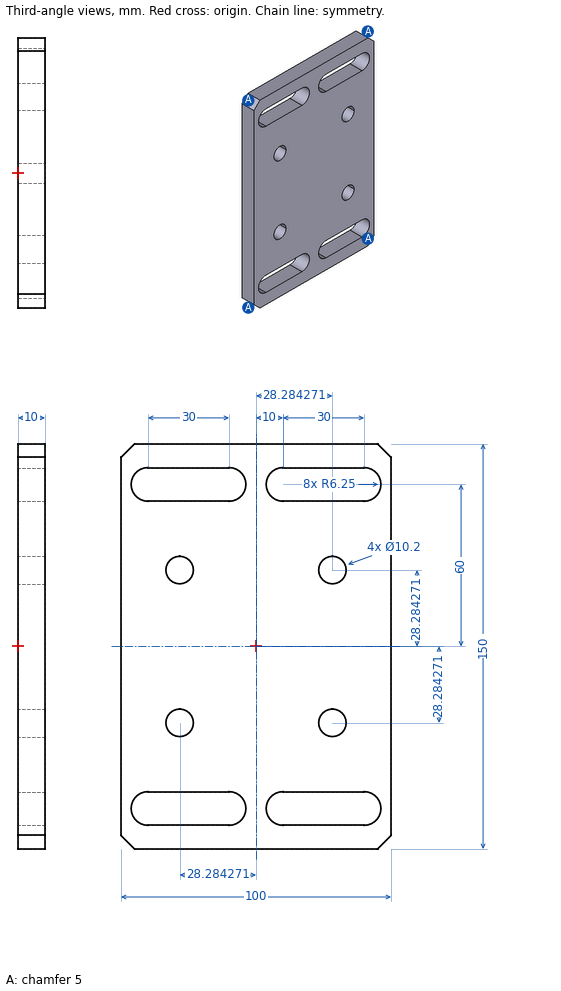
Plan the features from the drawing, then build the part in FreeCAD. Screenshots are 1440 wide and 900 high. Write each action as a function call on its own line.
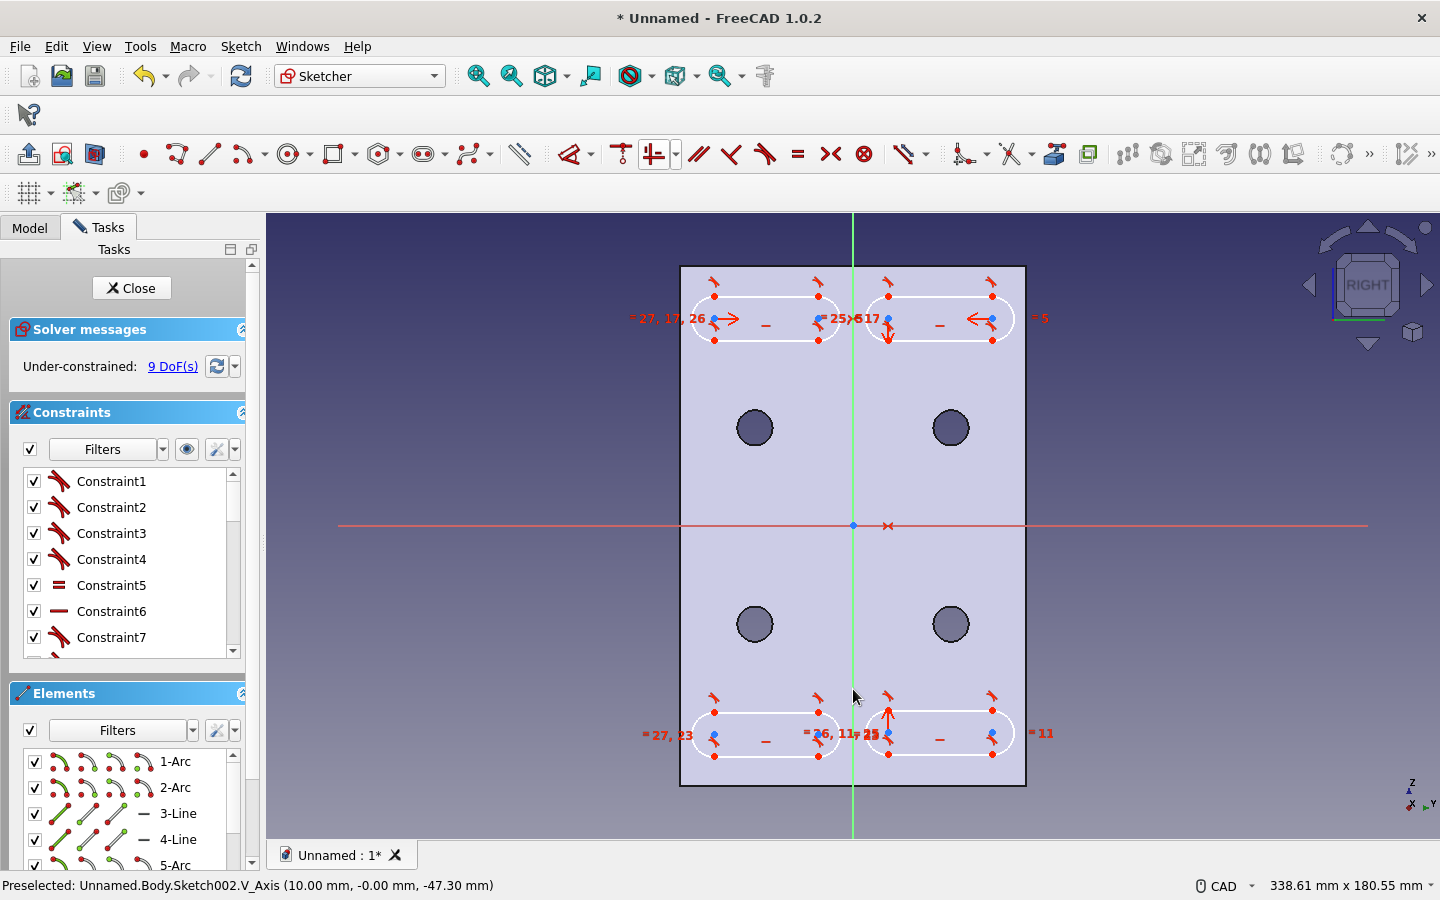
click(992, 733)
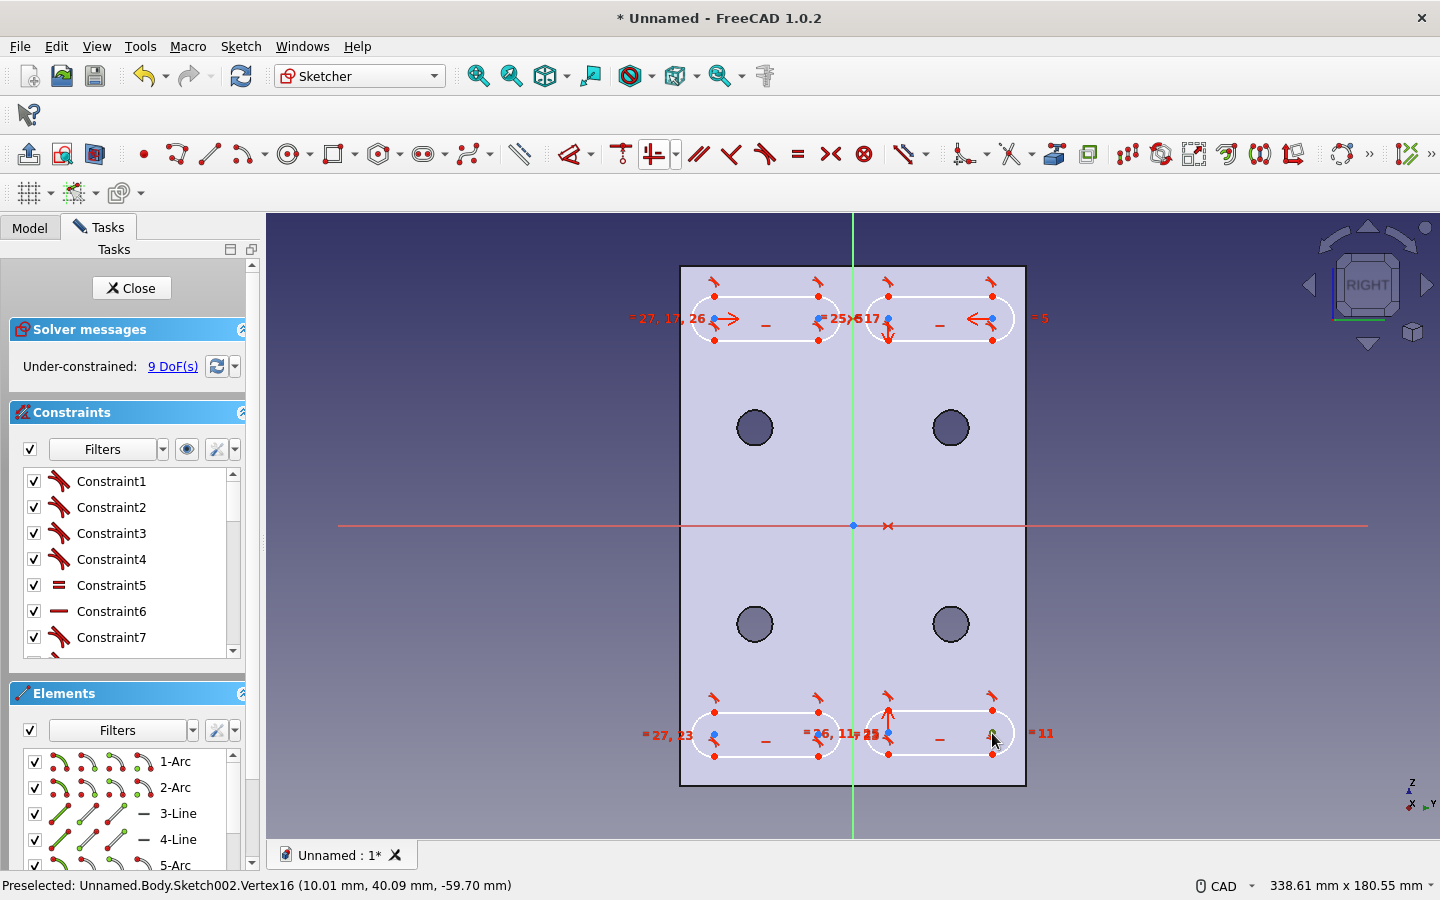
click(714, 735)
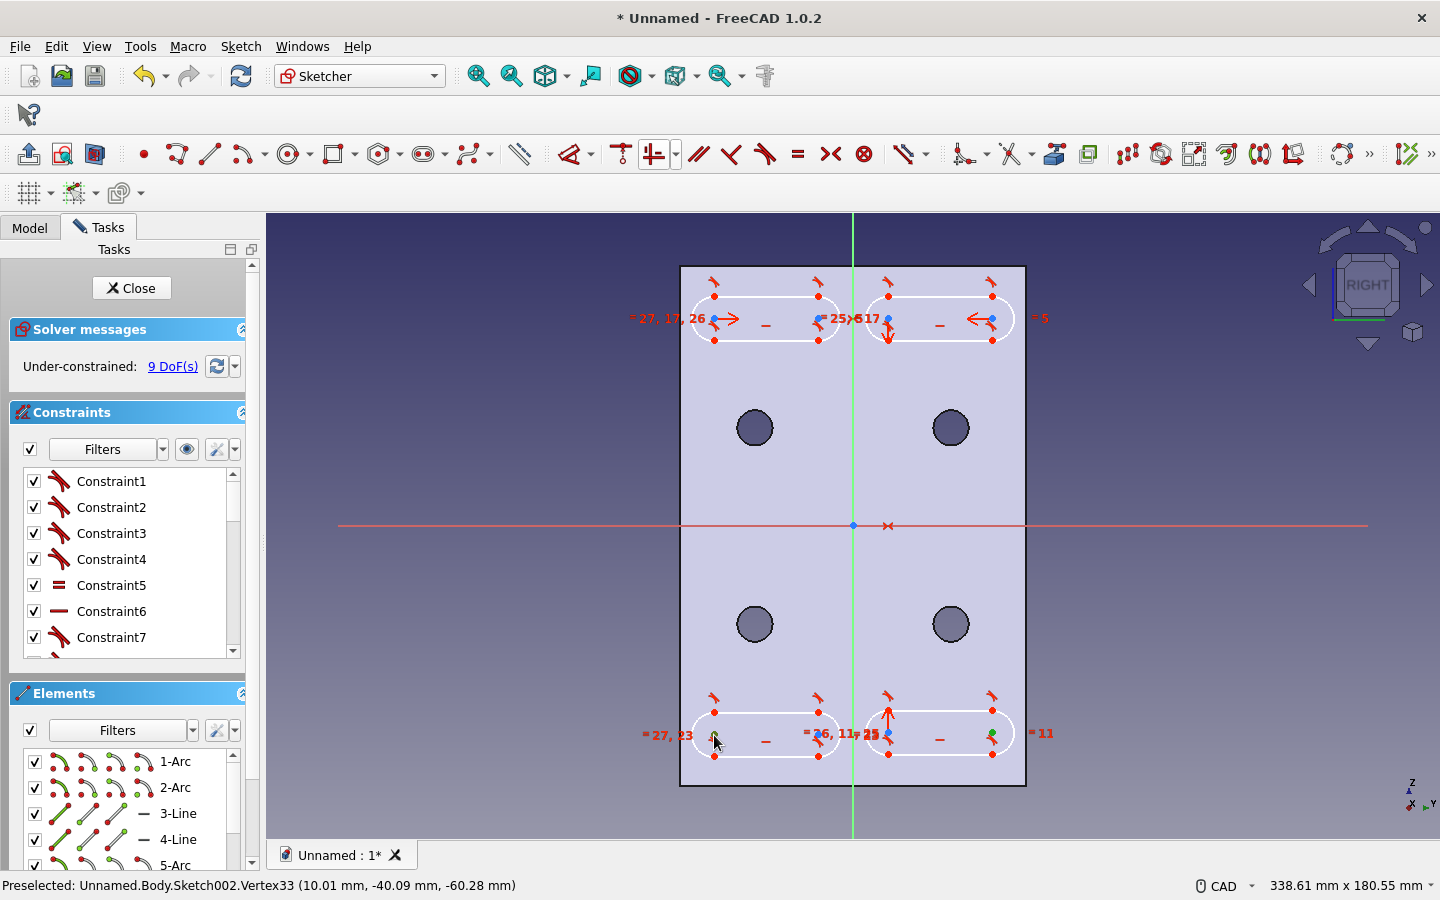
click(853, 689)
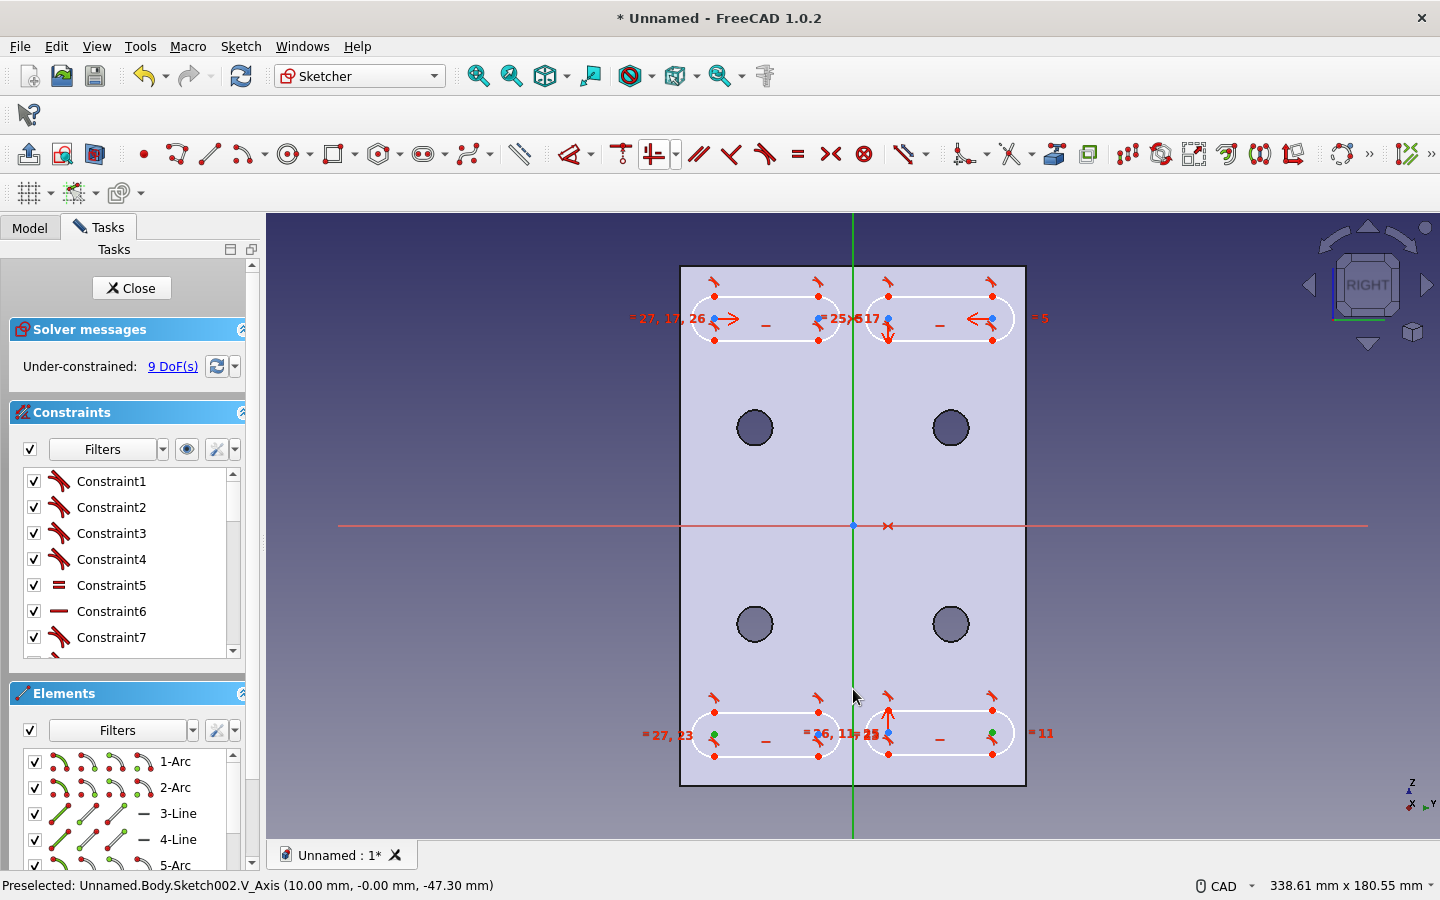
click(831, 154)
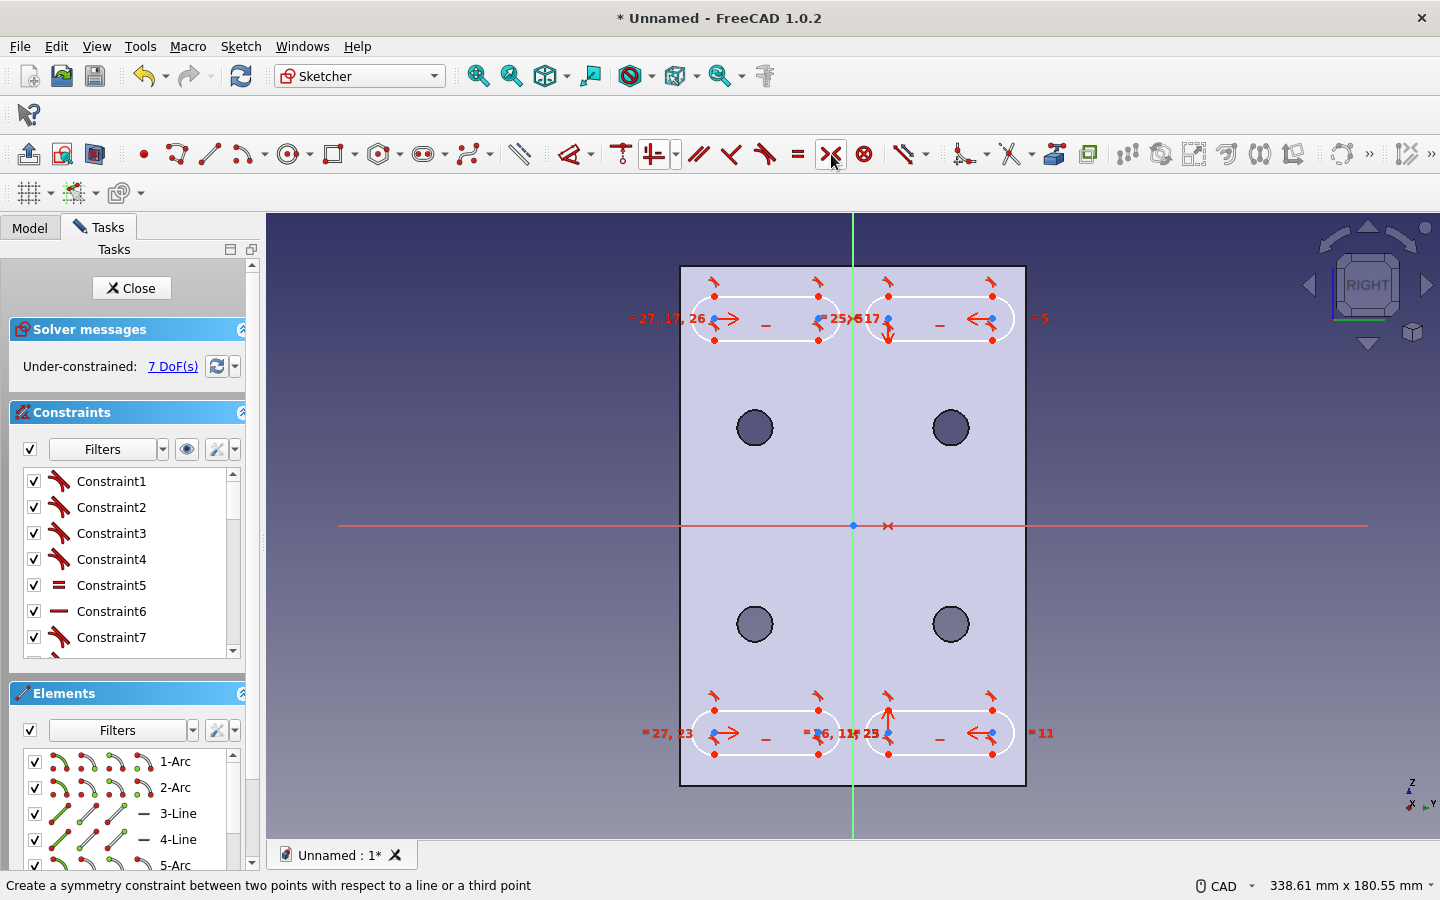
click(568, 154)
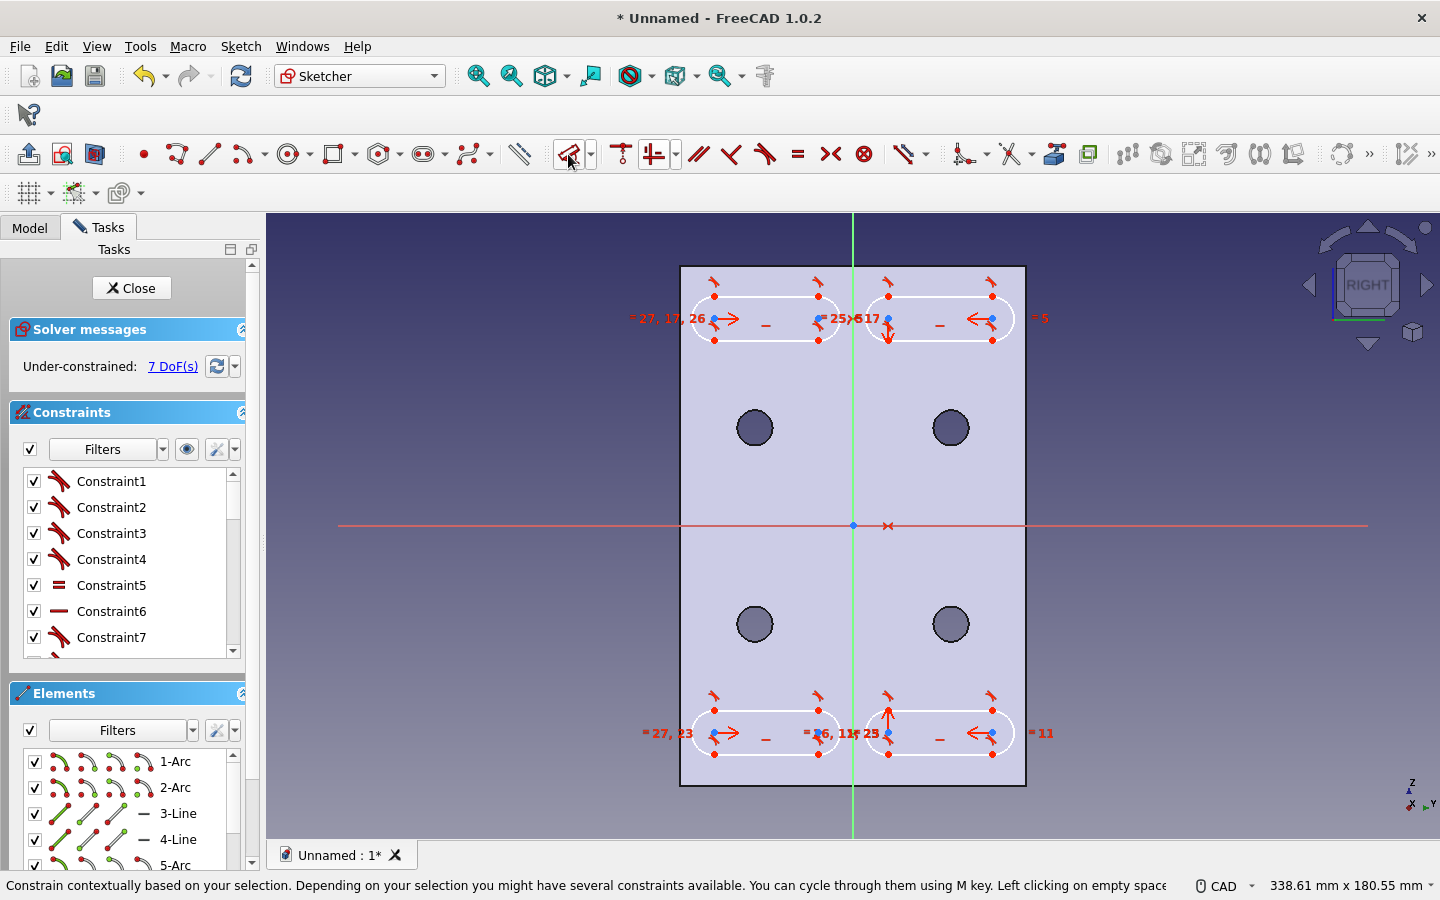
scroll(870, 306, up, 4)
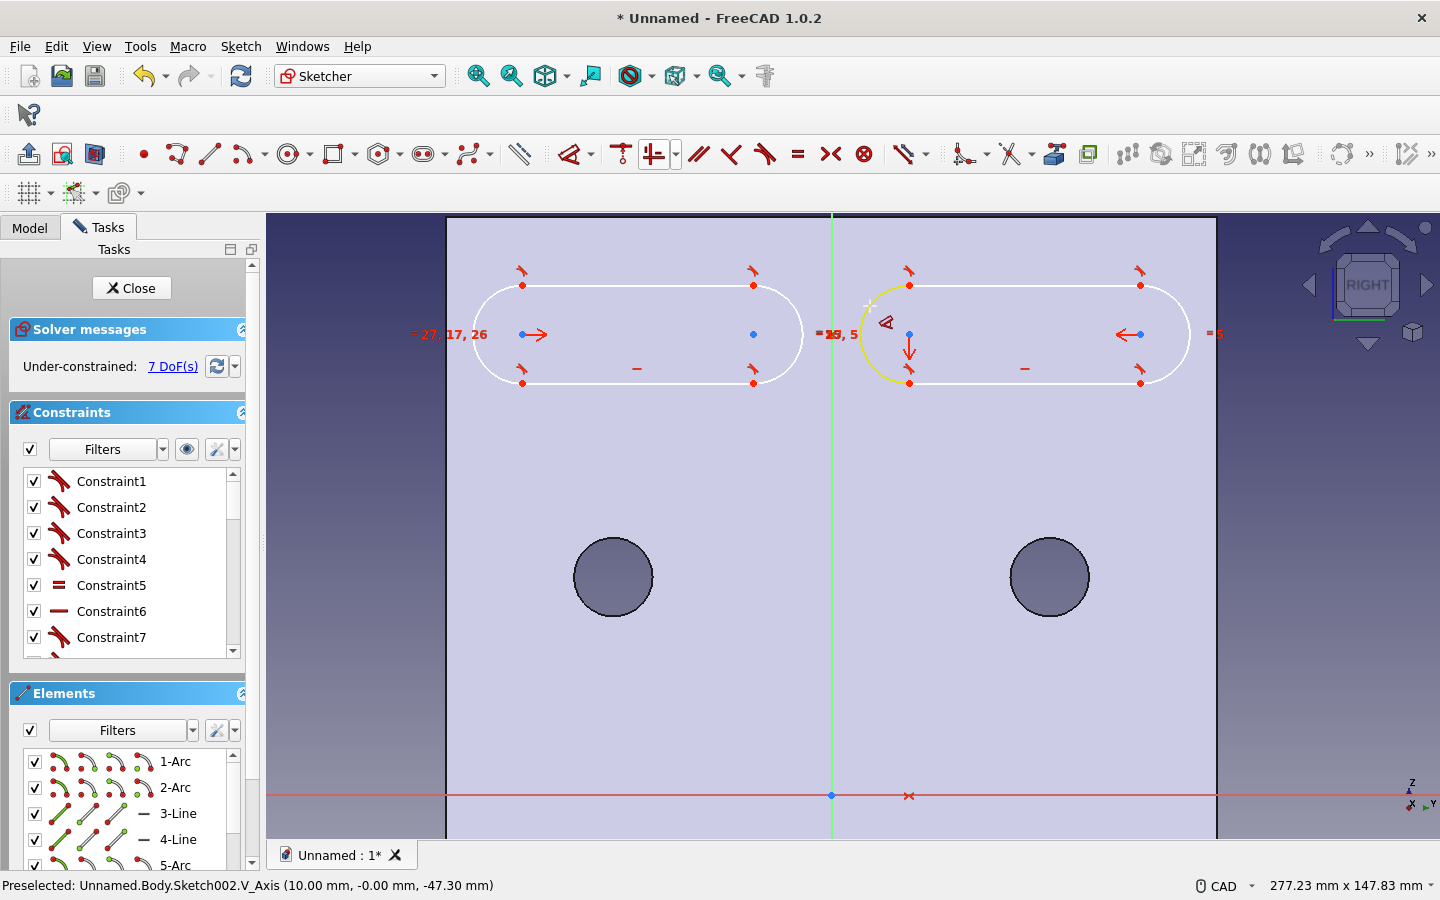
click(870, 306)
click(875, 262)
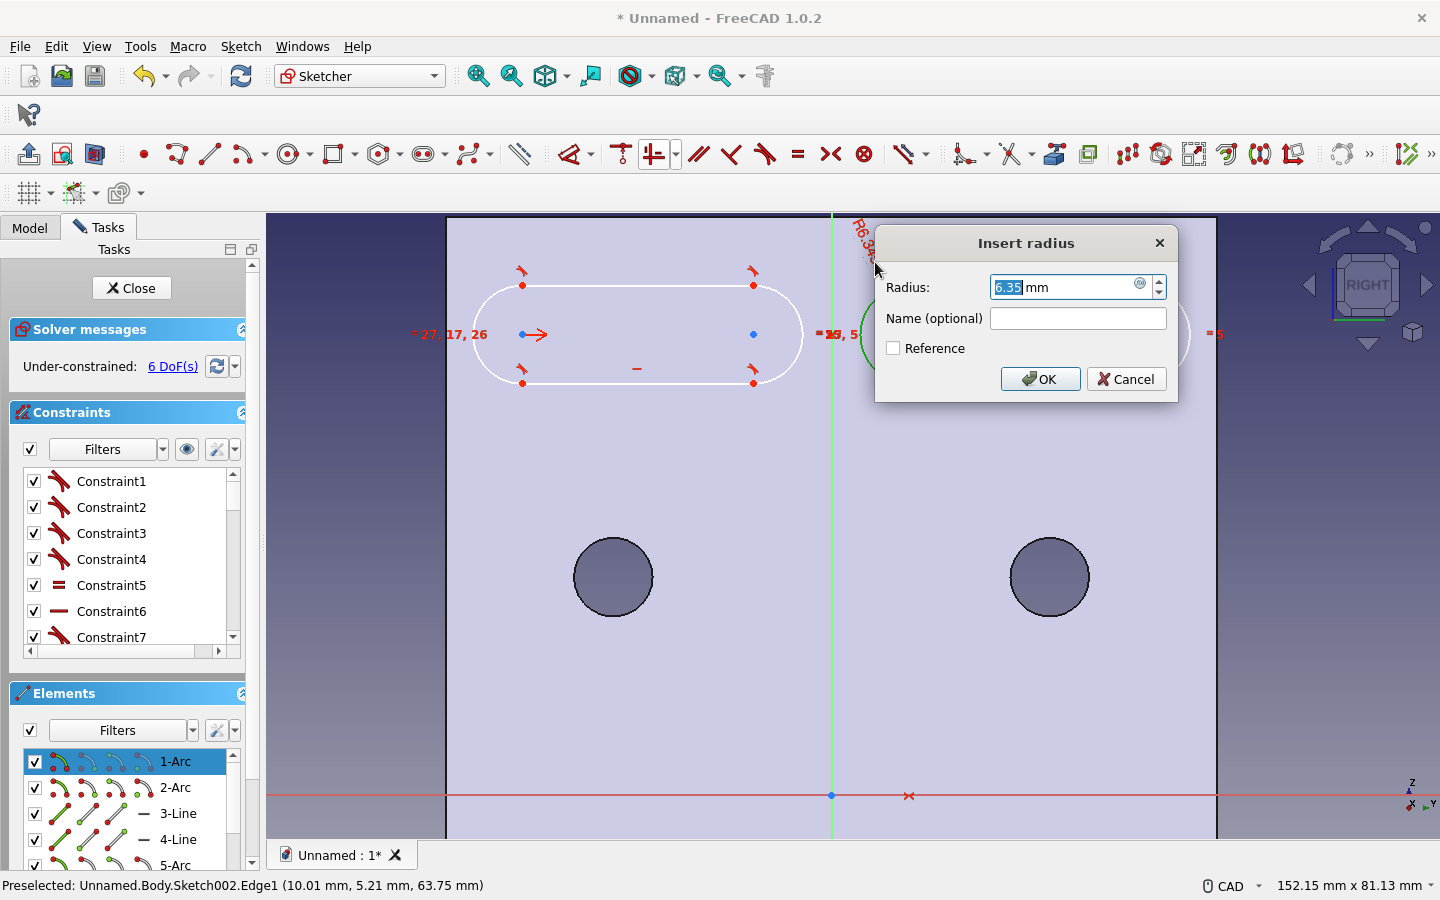
text(6.25)
key(Return)